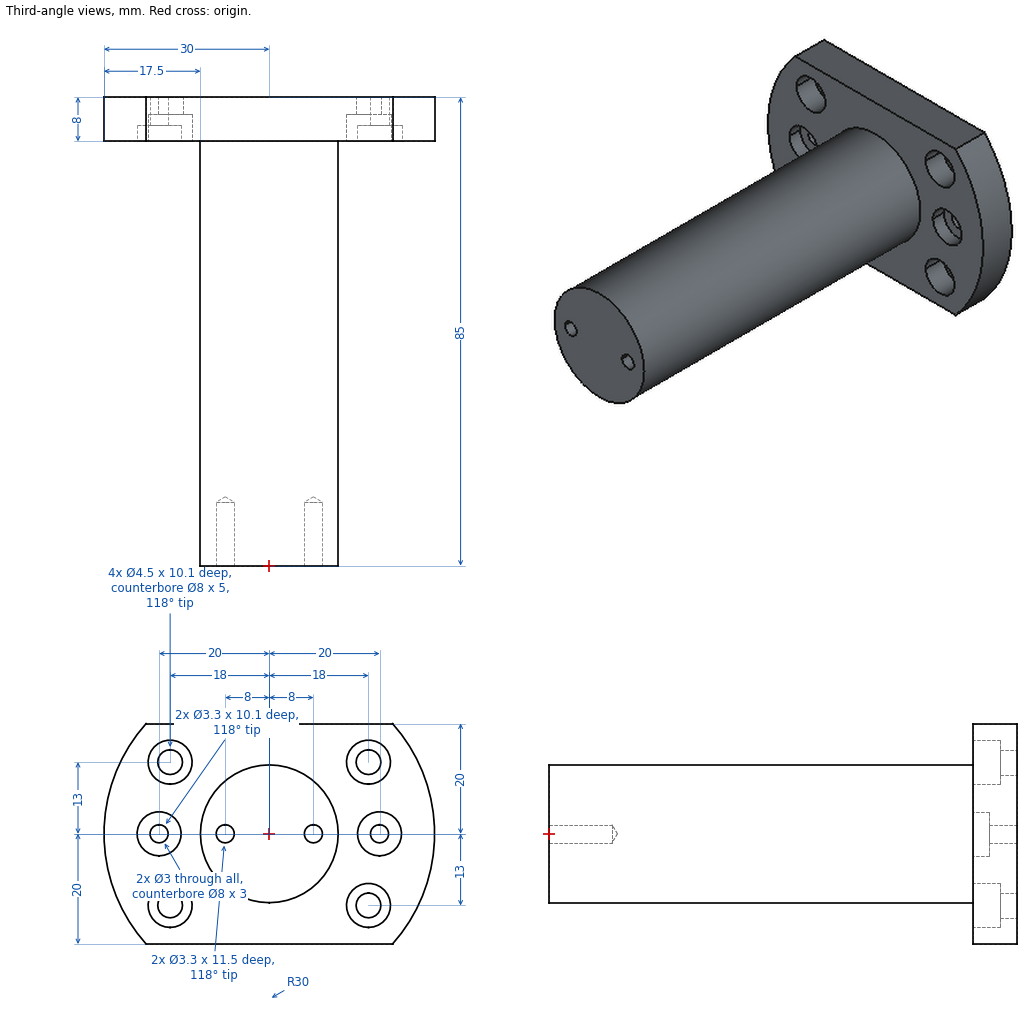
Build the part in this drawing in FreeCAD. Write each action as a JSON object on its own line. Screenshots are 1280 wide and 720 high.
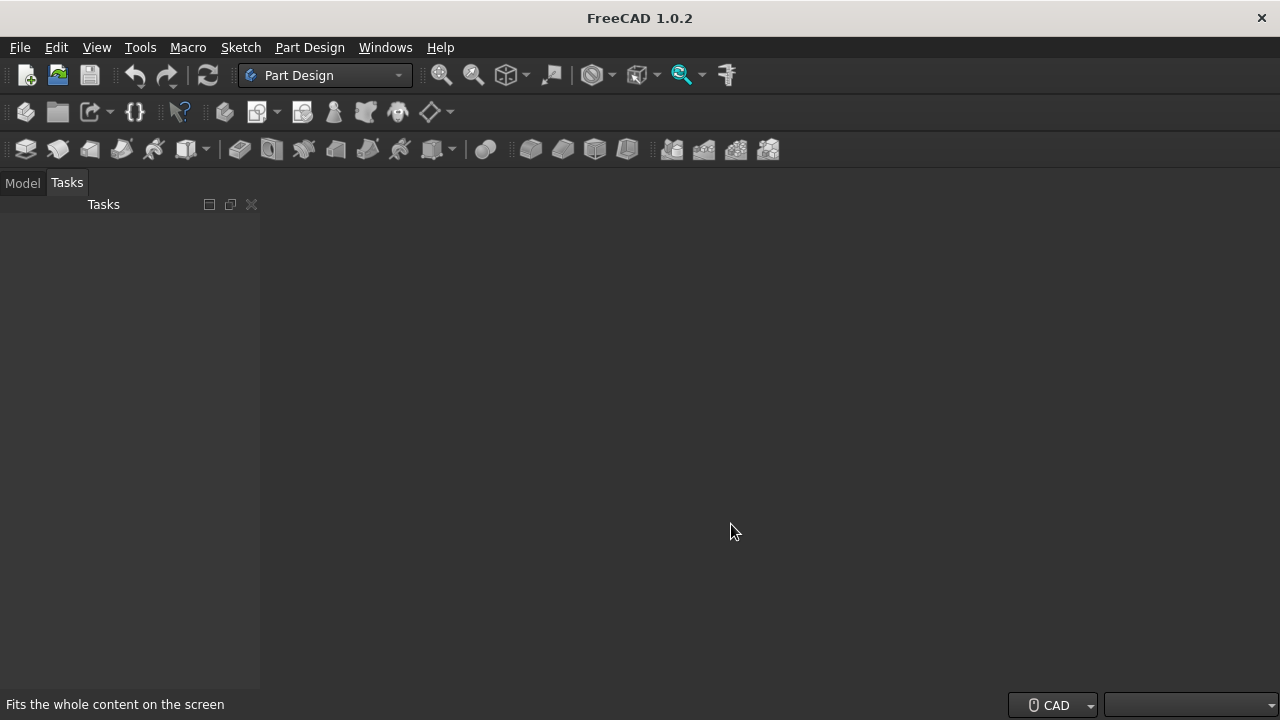
{"action": "left_click", "coordinate": [26, 76]}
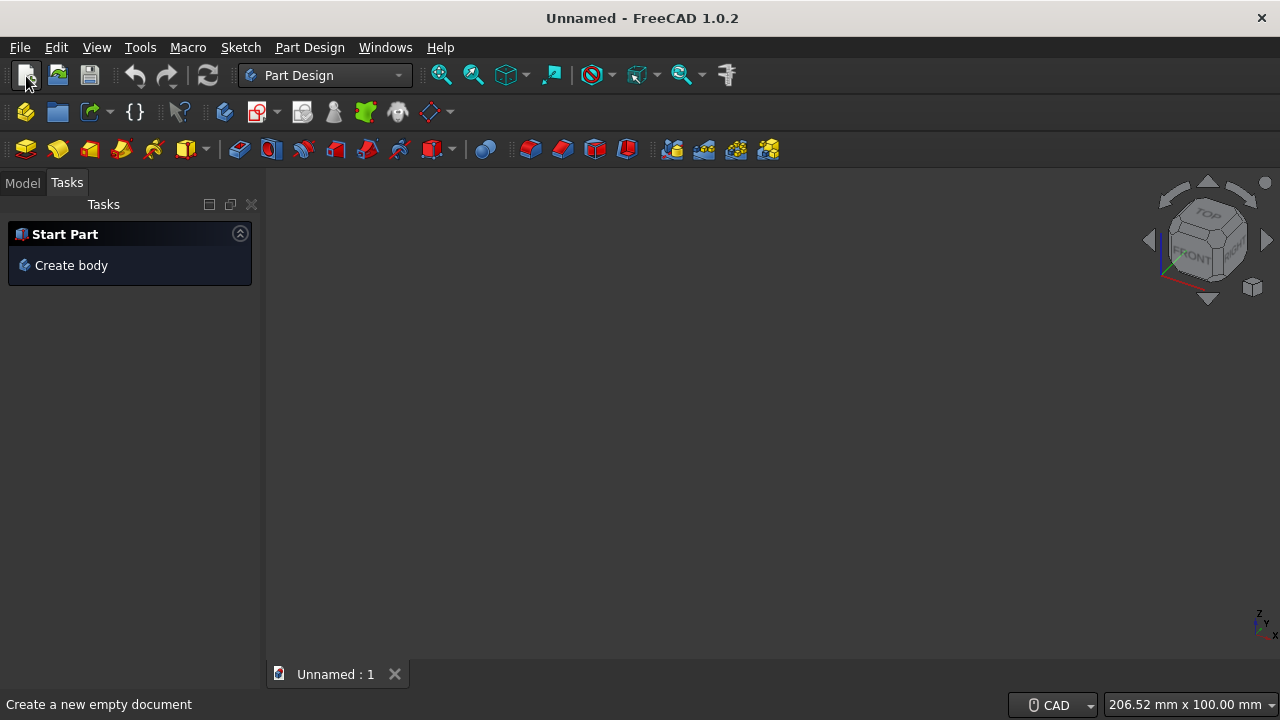
{"action": "left_click", "coordinate": [258, 112]}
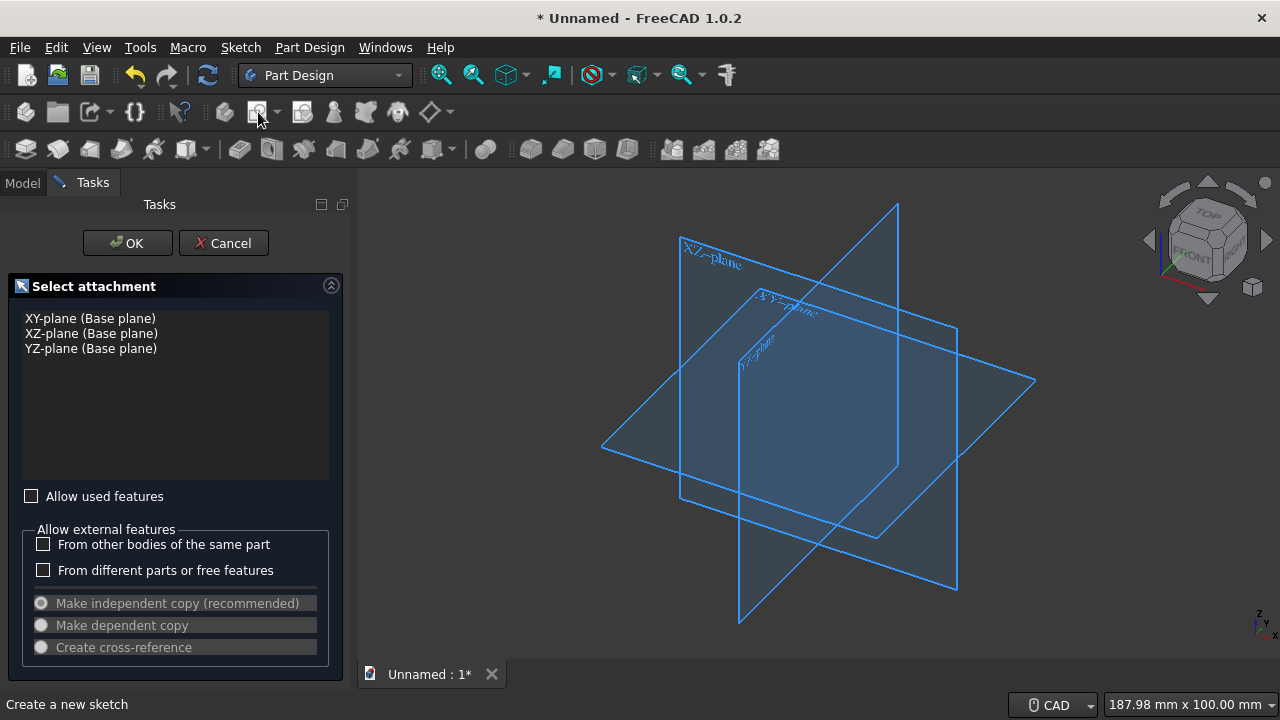
{"action": "left_click", "coordinate": [82, 318]}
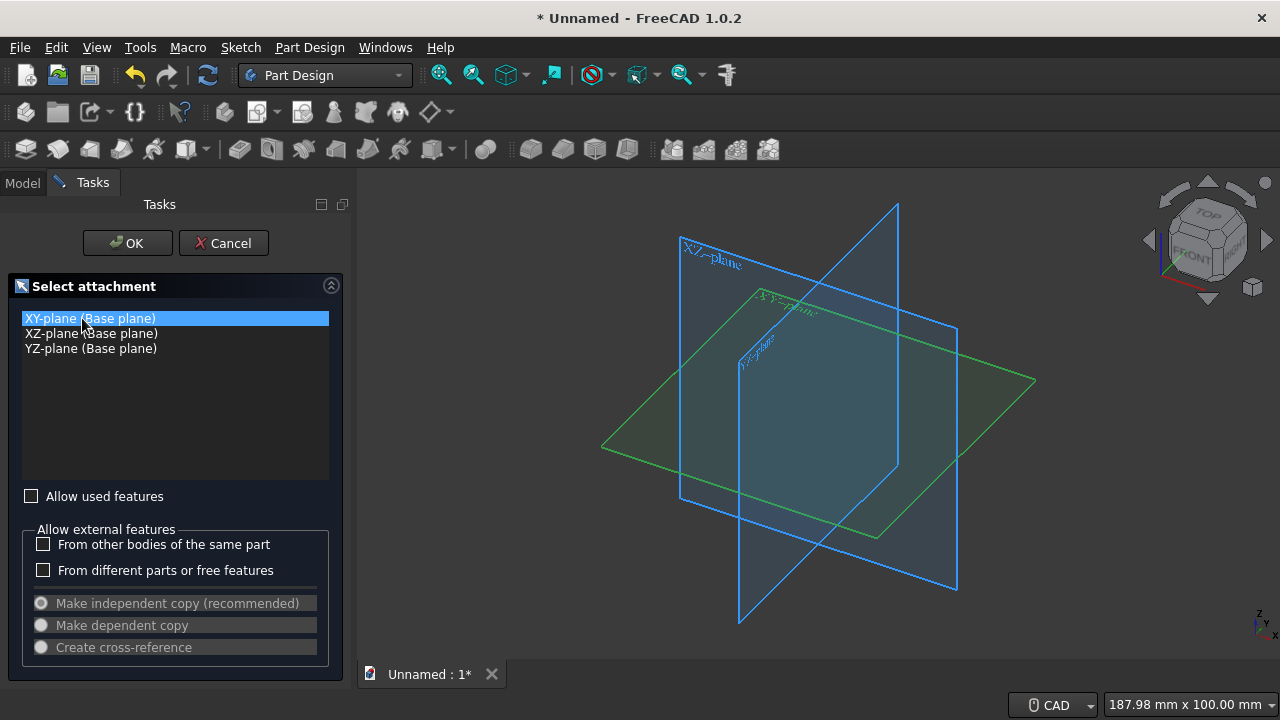
{"action": "left_click", "coordinate": [128, 243]}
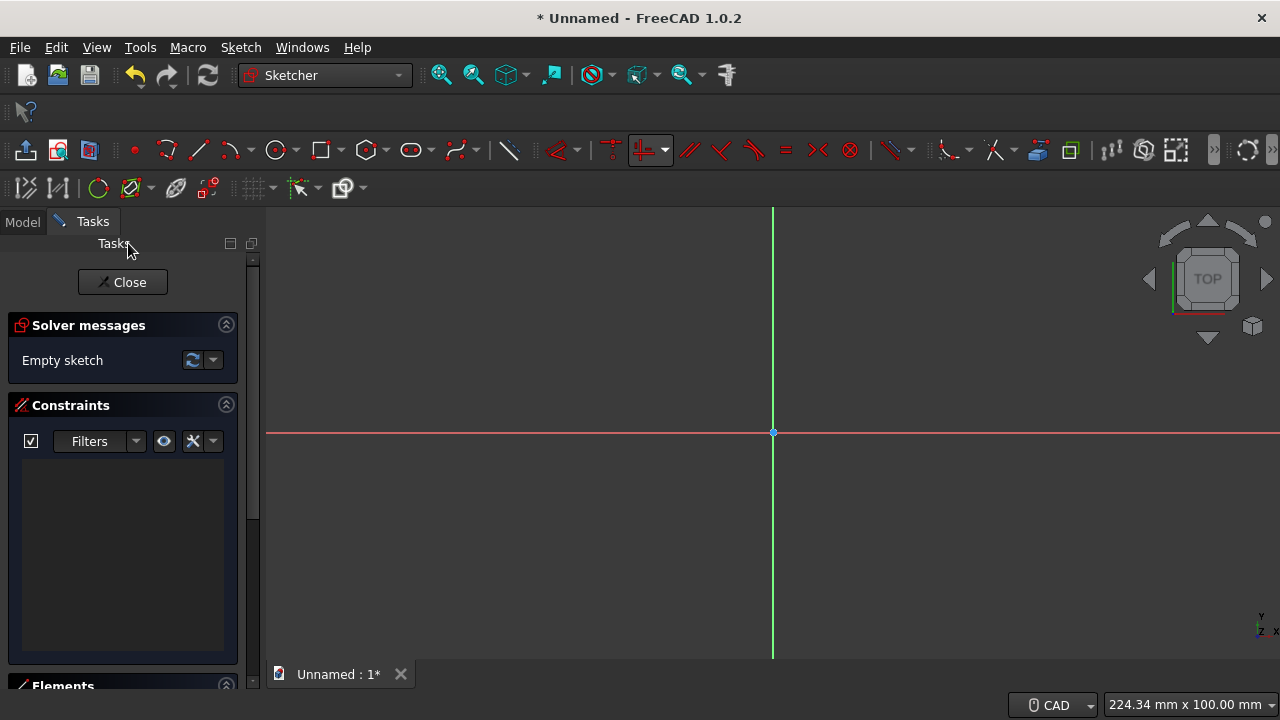
{"action": "scroll", "coordinate": [704, 631], "scroll_direction": "down", "scroll_amount": 3}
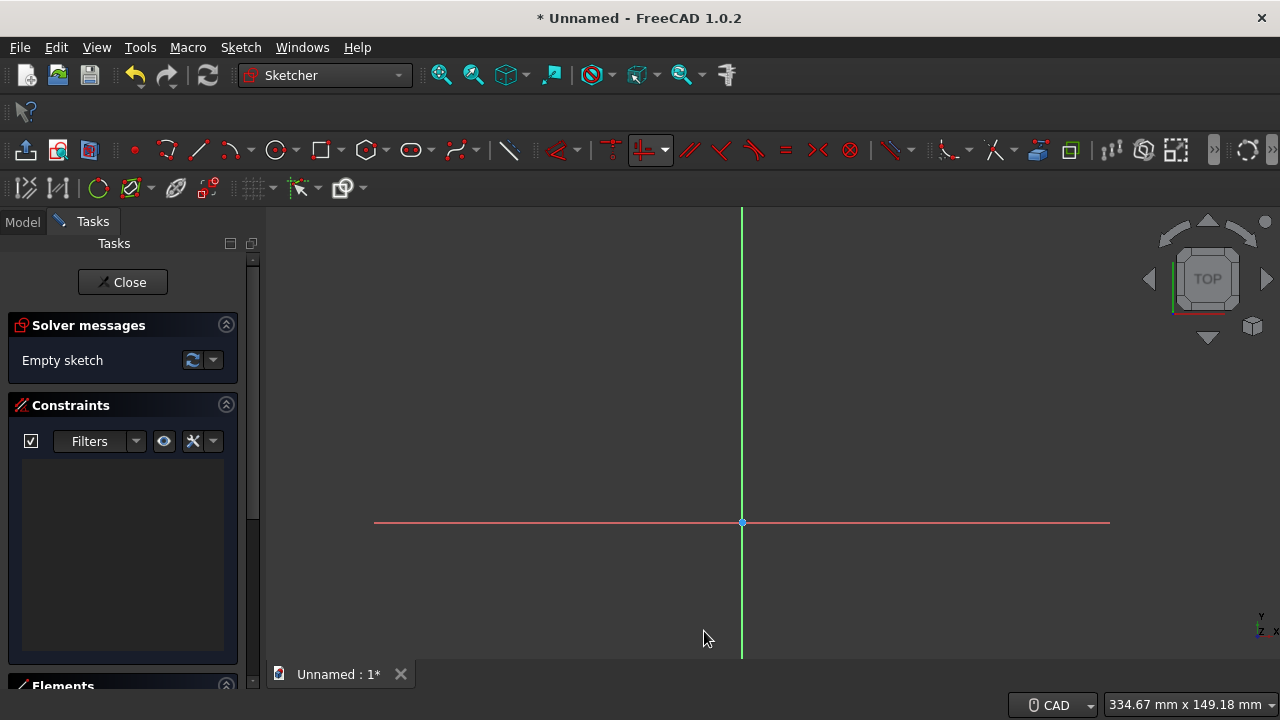
{"action": "left_click", "coordinate": [168, 150]}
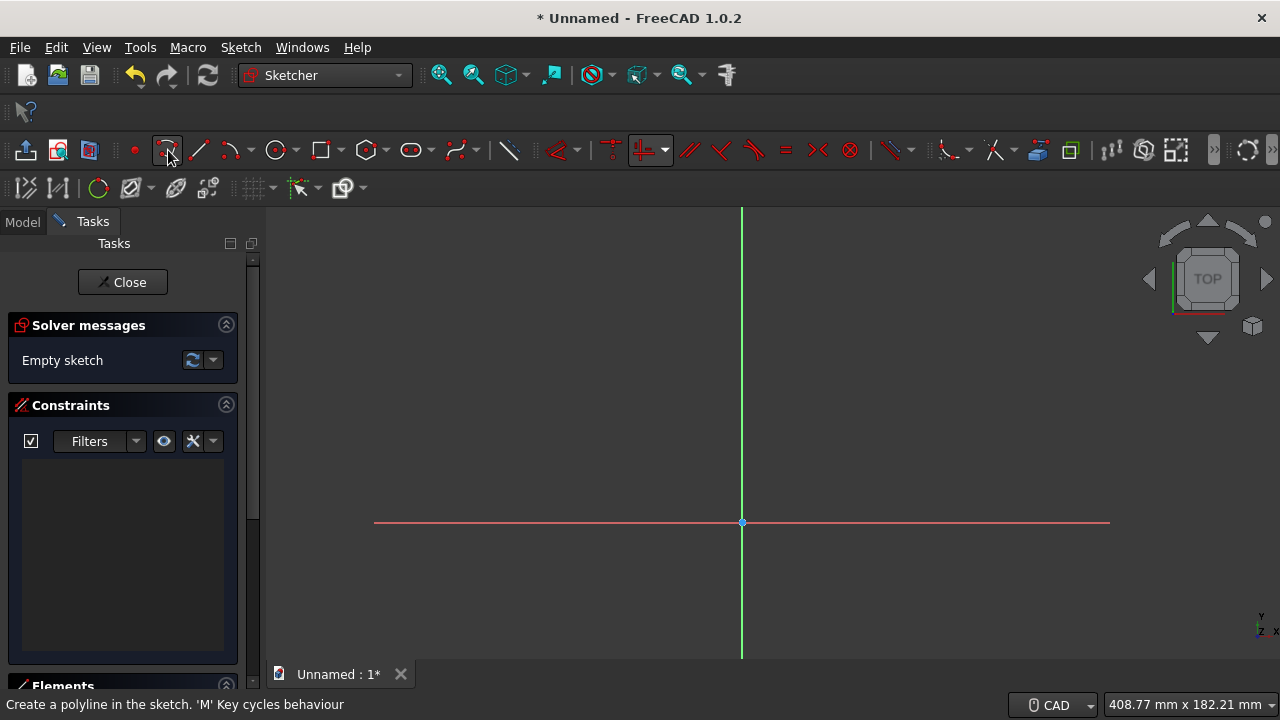
{"action": "left_click", "coordinate": [742, 523]}
{"action": "left_click", "coordinate": [733, 312]}
{"action": "left_click", "coordinate": [668, 312]}
{"action": "left_click", "coordinate": [668, 332]}
{"action": "left_click", "coordinate": [711, 332]}
{"action": "left_click", "coordinate": [711, 514]}
{"action": "left_click", "coordinate": [742, 523]}
{"action": "key", "text": "Escape"}
{"action": "key", "text": "Escape"}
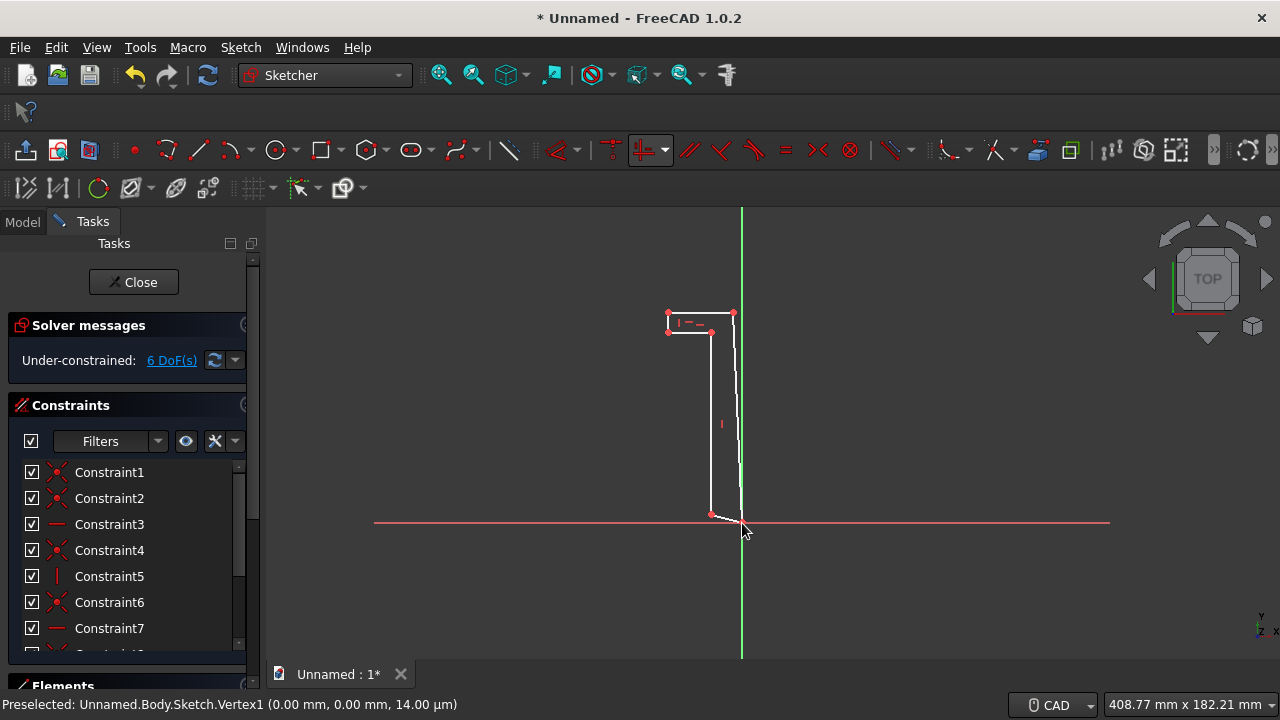
{"action": "left_click", "coordinate": [739, 460]}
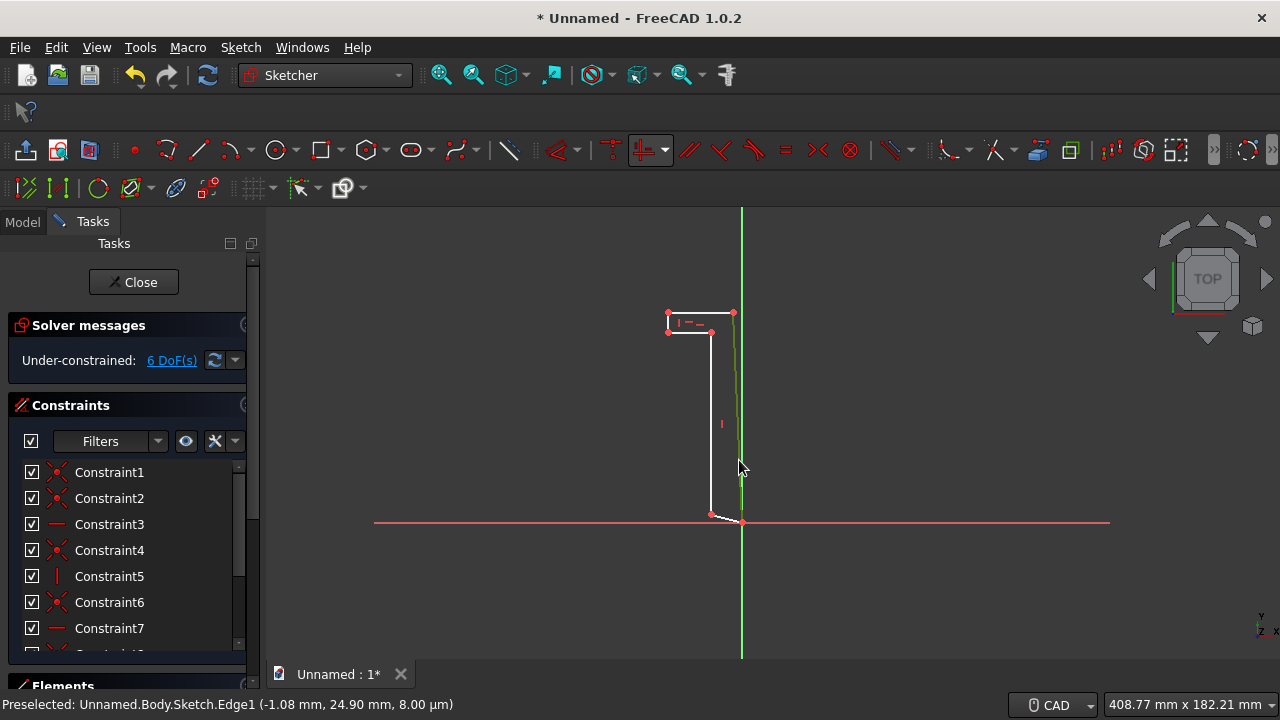
{"action": "left_click", "coordinate": [668, 150]}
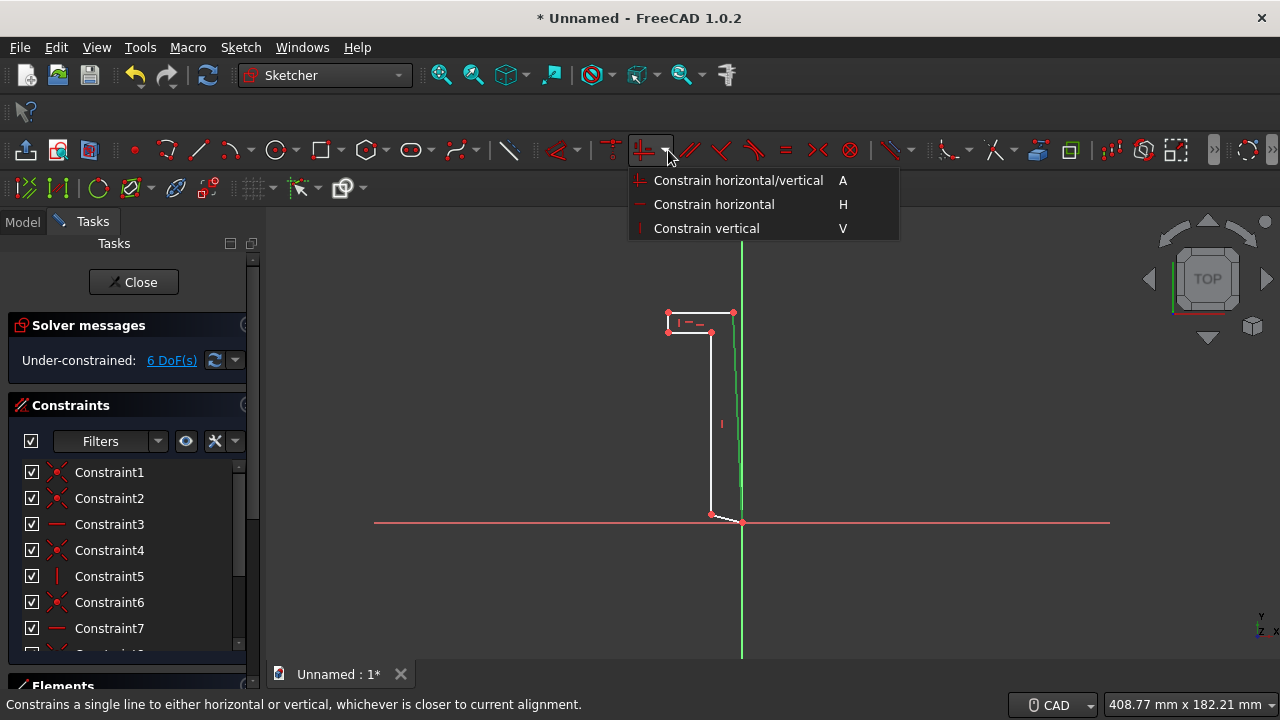
{"action": "left_click", "coordinate": [764, 228]}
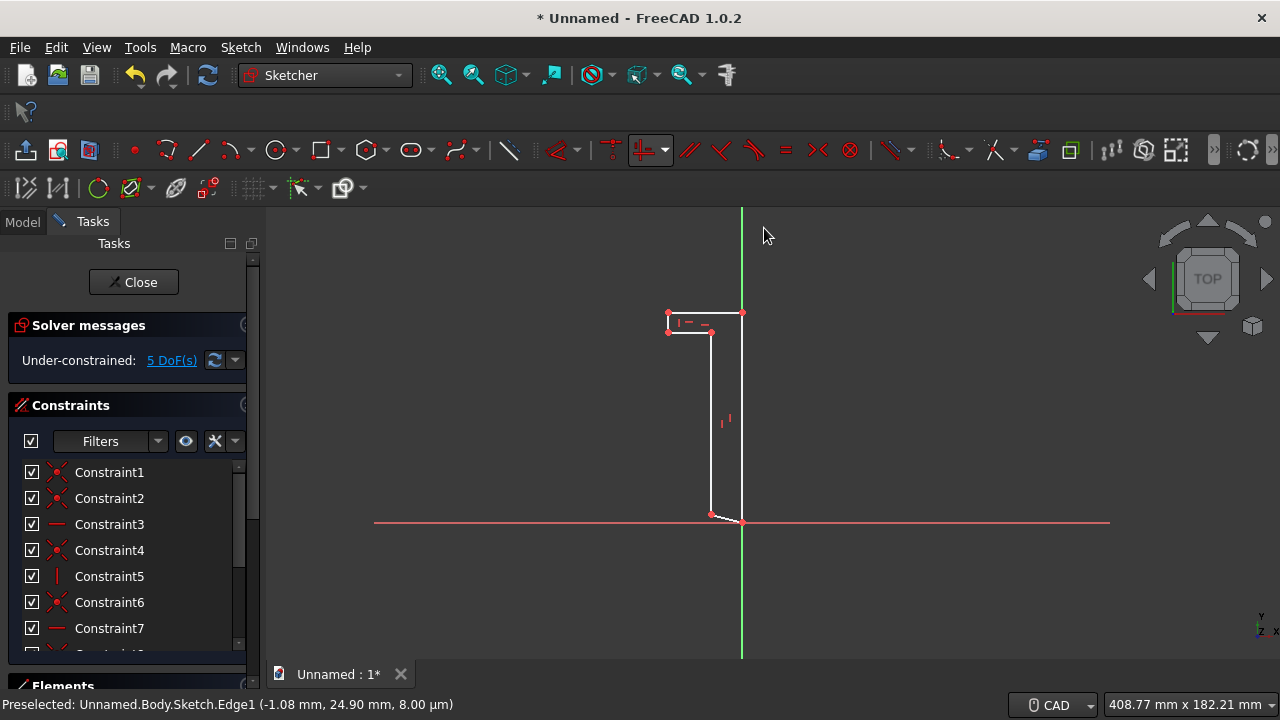
{"action": "scroll", "coordinate": [733, 520], "scroll_direction": "up", "scroll_amount": 2}